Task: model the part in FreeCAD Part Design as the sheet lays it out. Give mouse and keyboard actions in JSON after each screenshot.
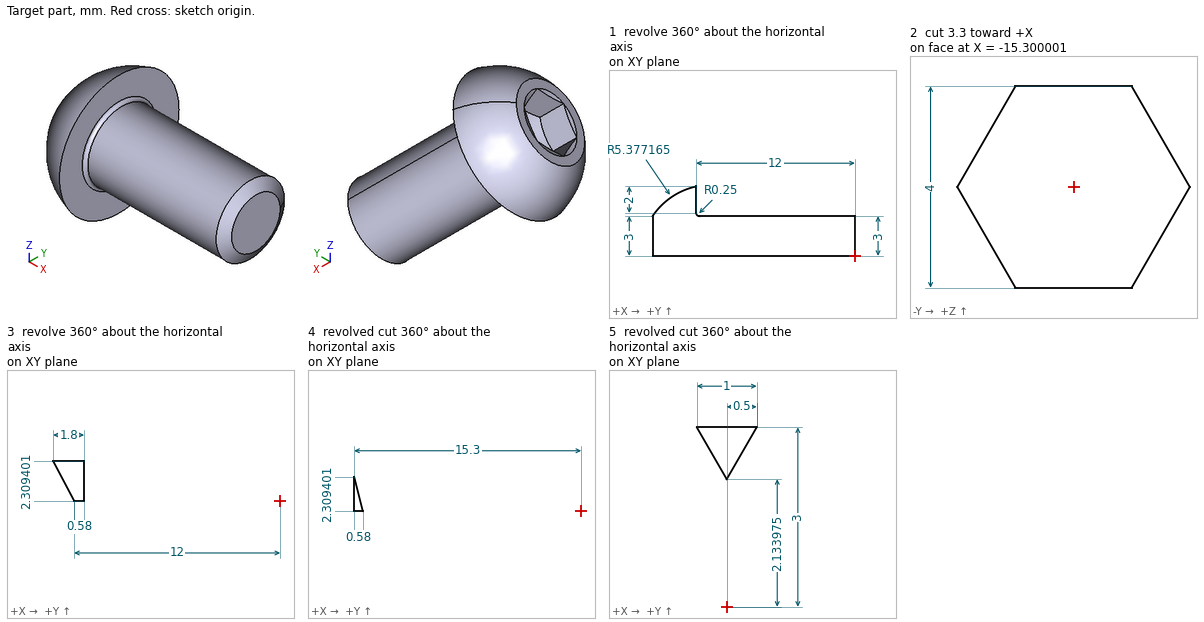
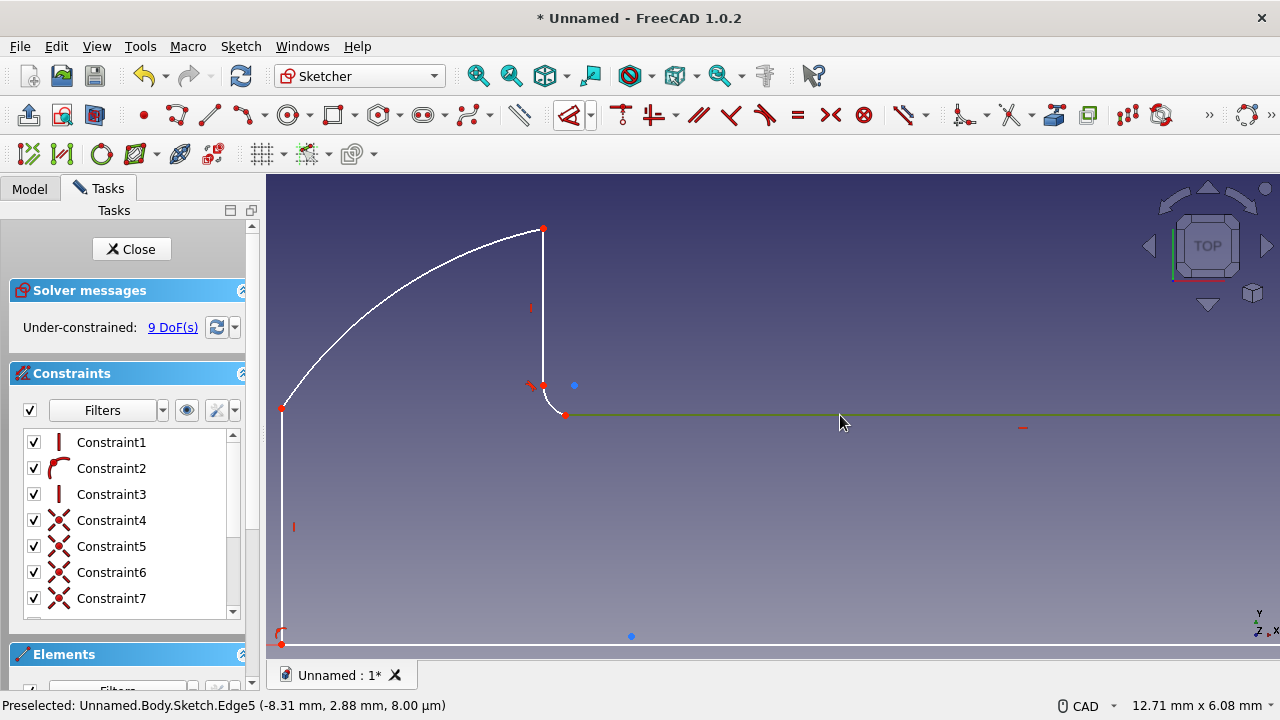
{"action": "left_click", "coordinate": [546, 397]}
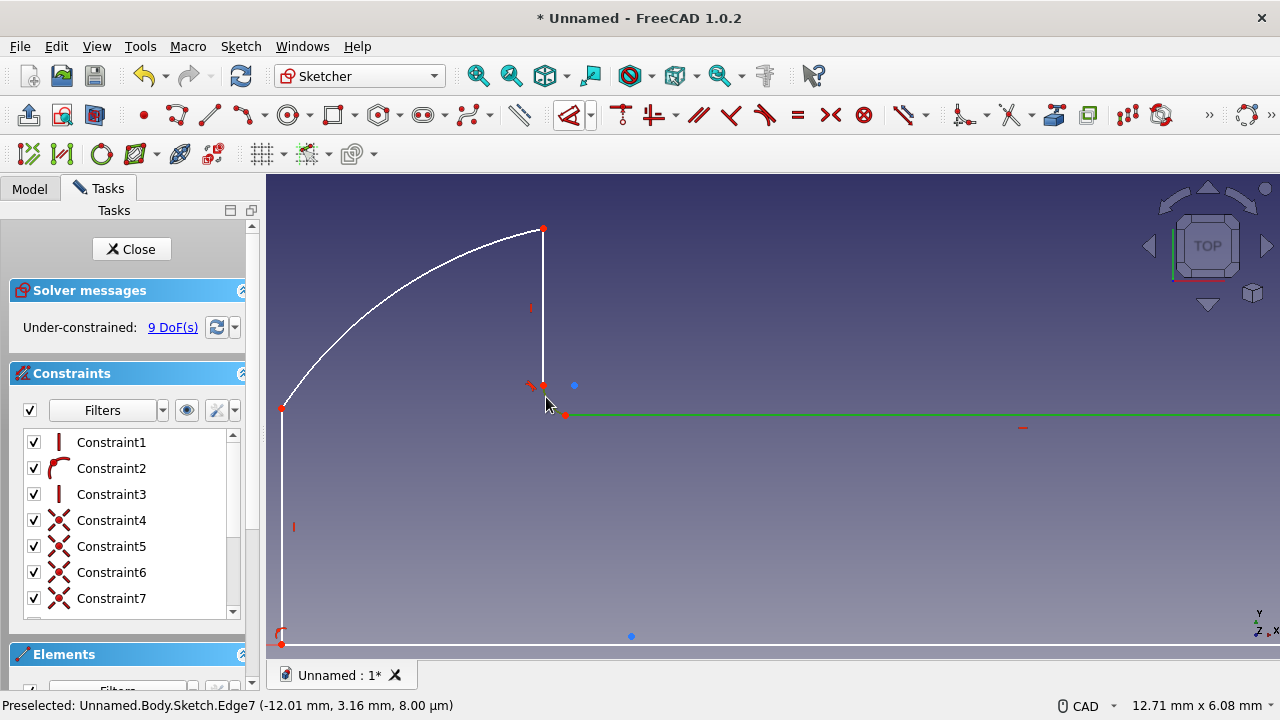
{"action": "left_click", "coordinate": [765, 116]}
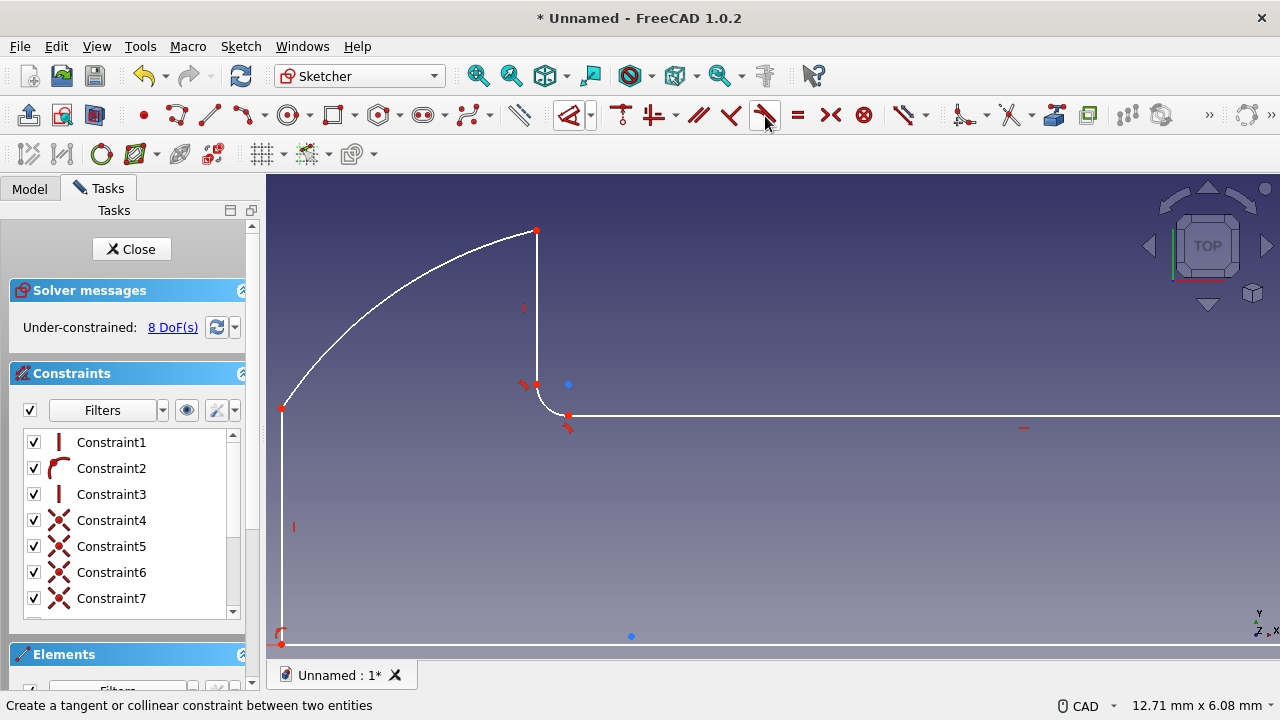
{"action": "scroll", "coordinate": [551, 401], "scroll_direction": "down", "scroll_amount": 4}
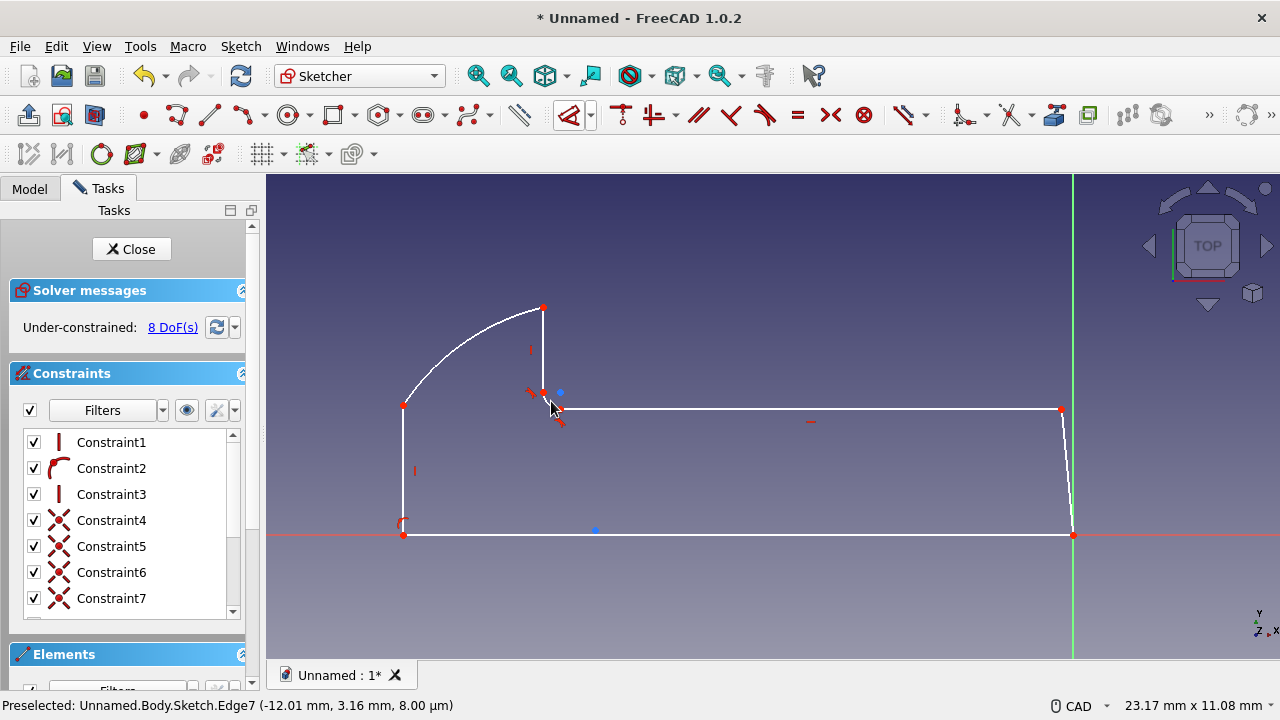
{"action": "scroll", "coordinate": [972, 439], "scroll_direction": "up", "scroll_amount": 4}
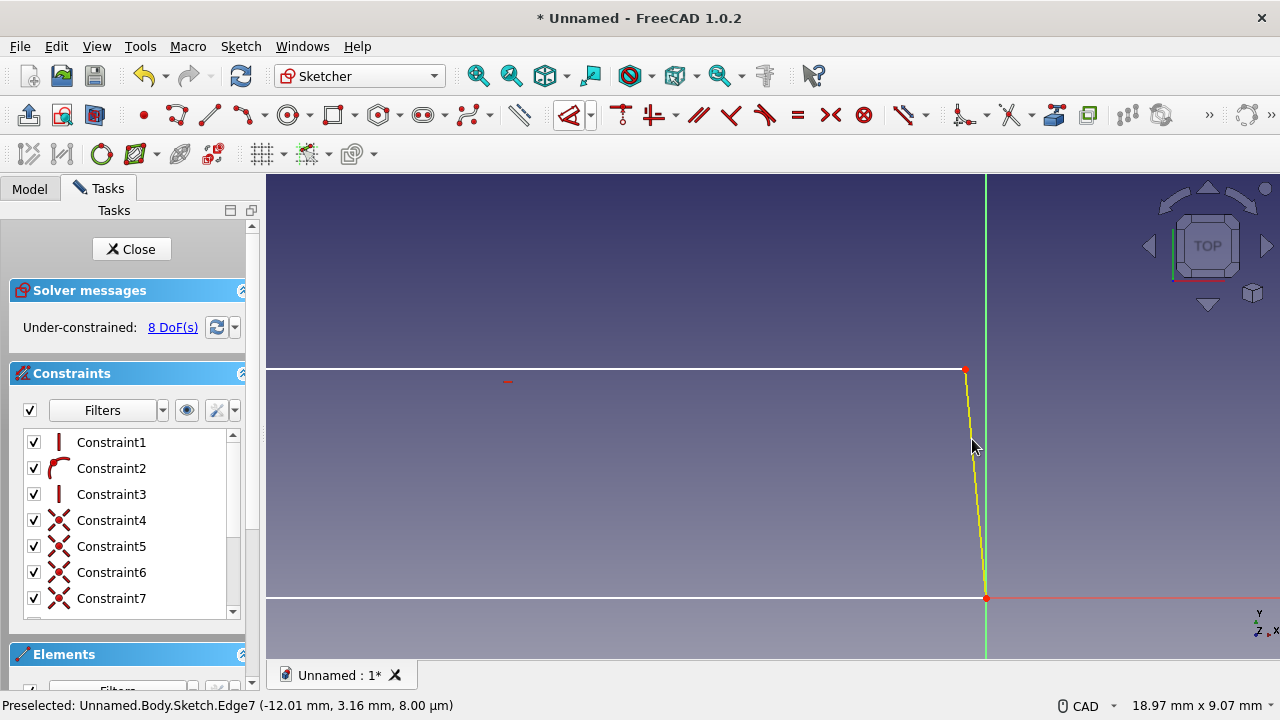
{"action": "left_click", "coordinate": [971, 438]}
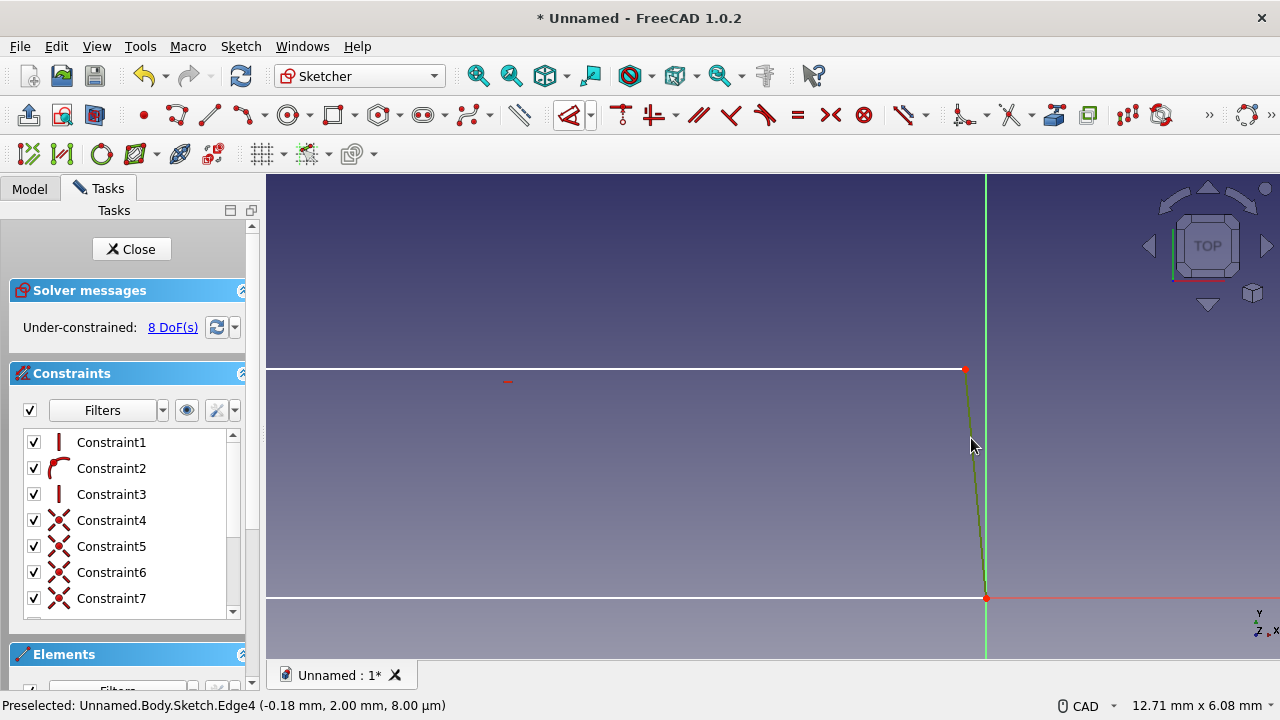
{"action": "key", "text": "v"}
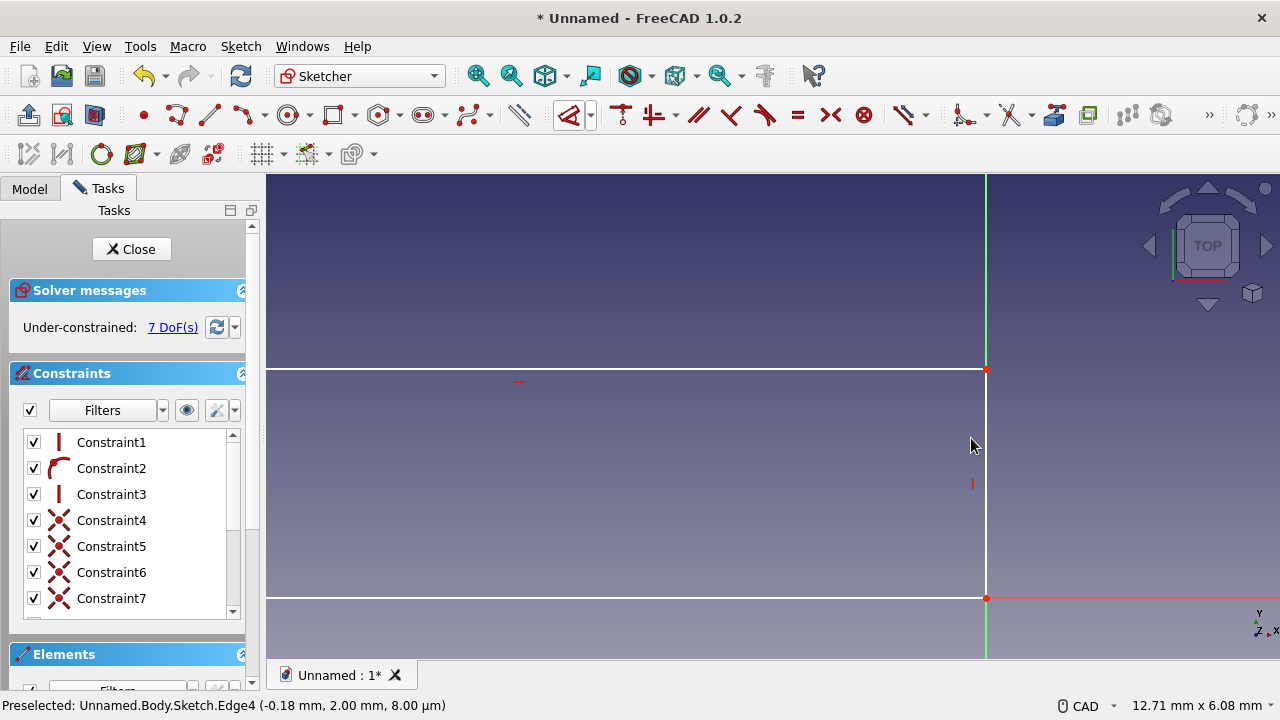
{"action": "scroll", "coordinate": [973, 439], "scroll_direction": "down", "scroll_amount": 4}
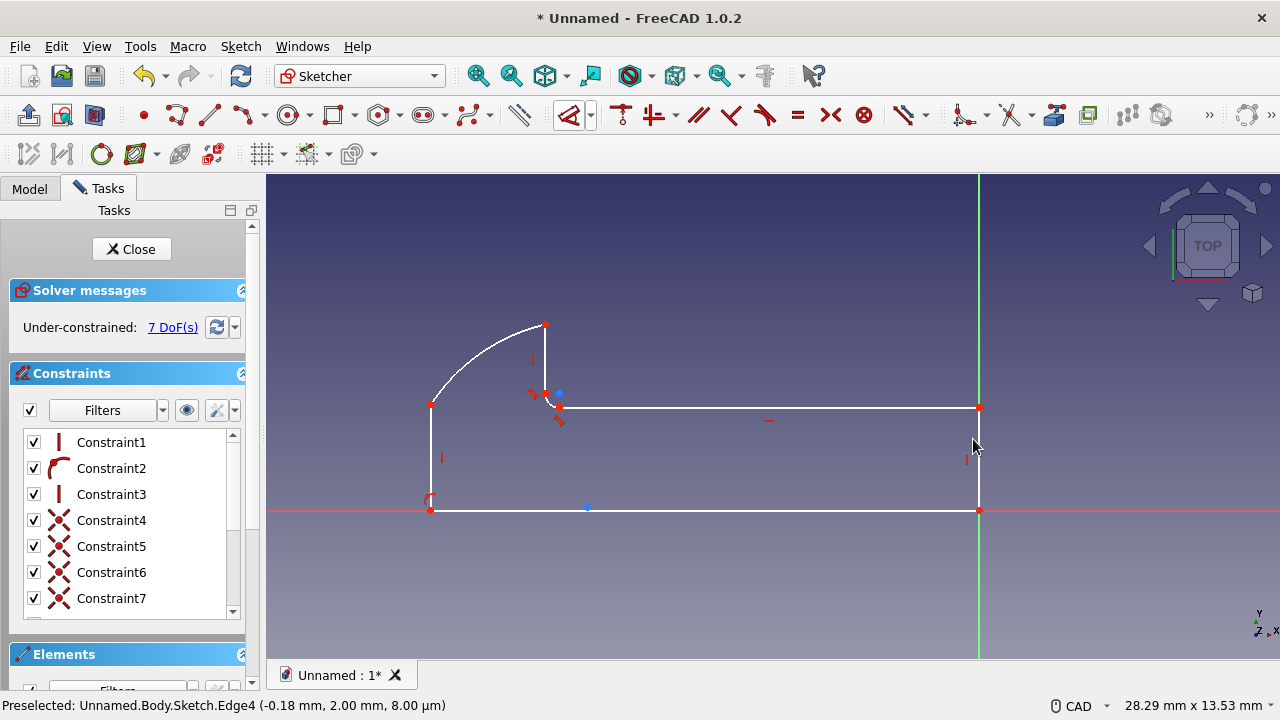
{"action": "left_click", "coordinate": [588, 507]}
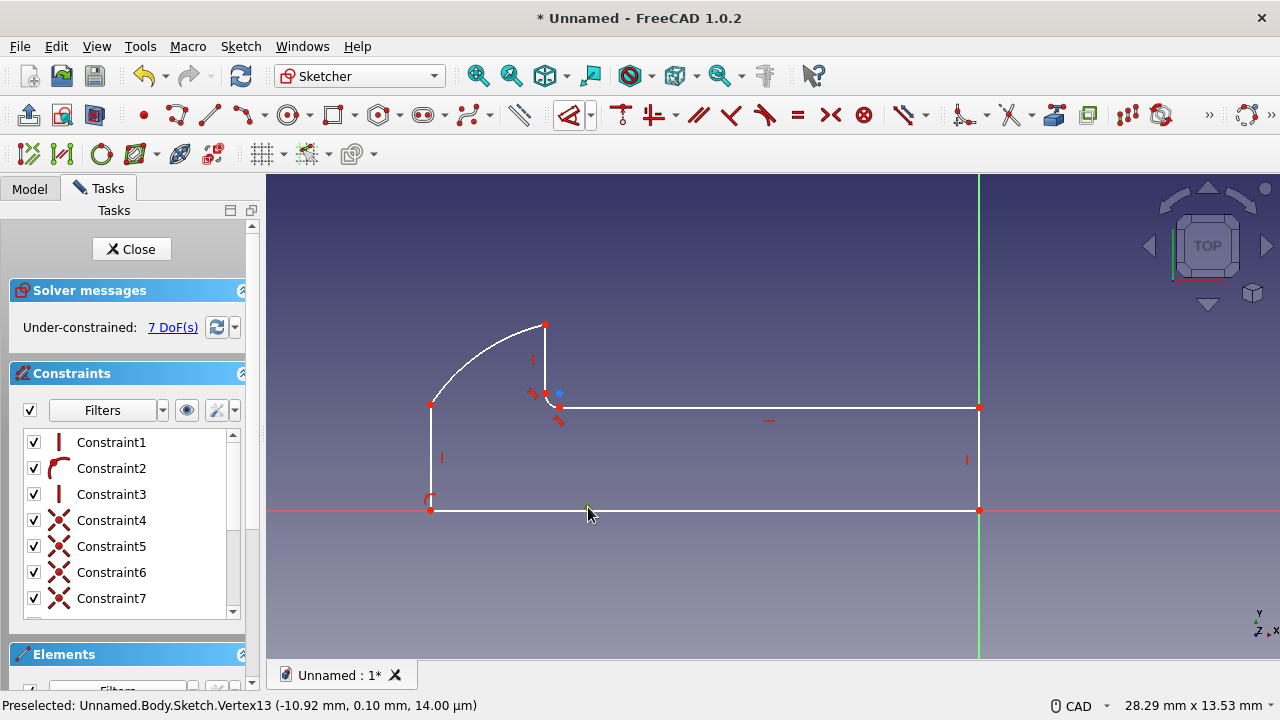
{"action": "left_click", "coordinate": [353, 511]}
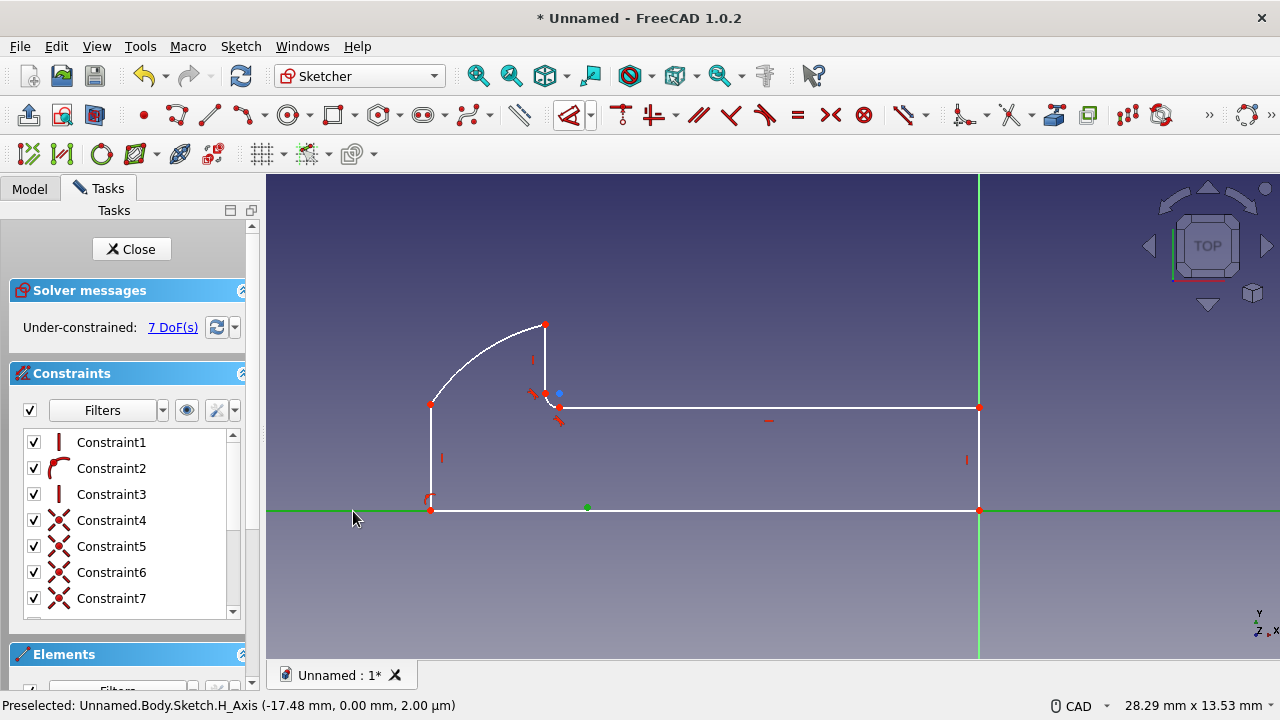
{"action": "left_click", "coordinate": [621, 116]}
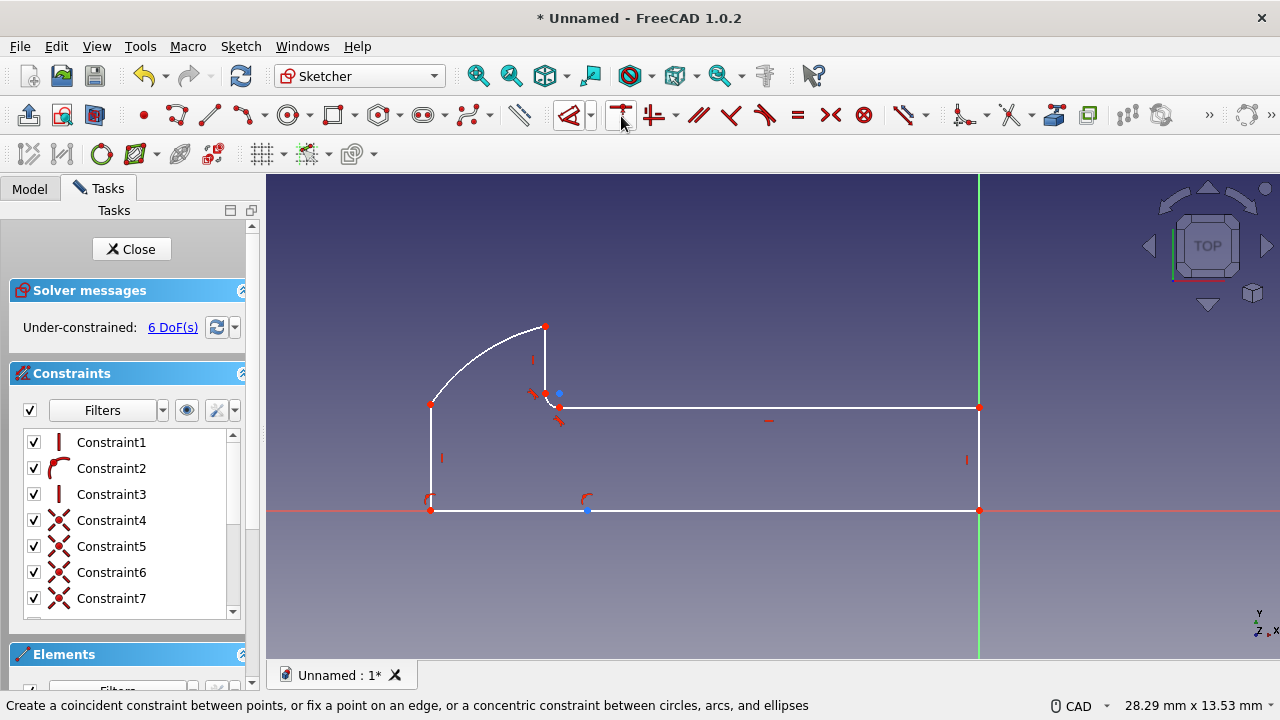
{"action": "left_click", "coordinate": [568, 116]}